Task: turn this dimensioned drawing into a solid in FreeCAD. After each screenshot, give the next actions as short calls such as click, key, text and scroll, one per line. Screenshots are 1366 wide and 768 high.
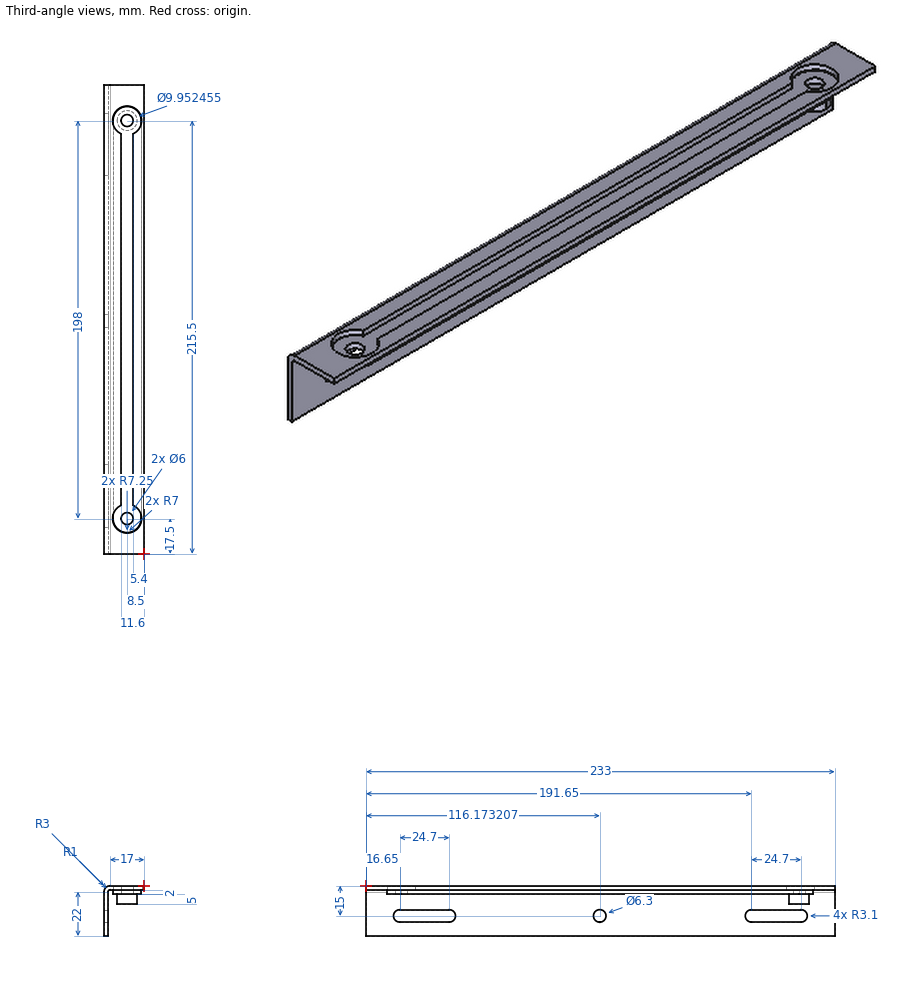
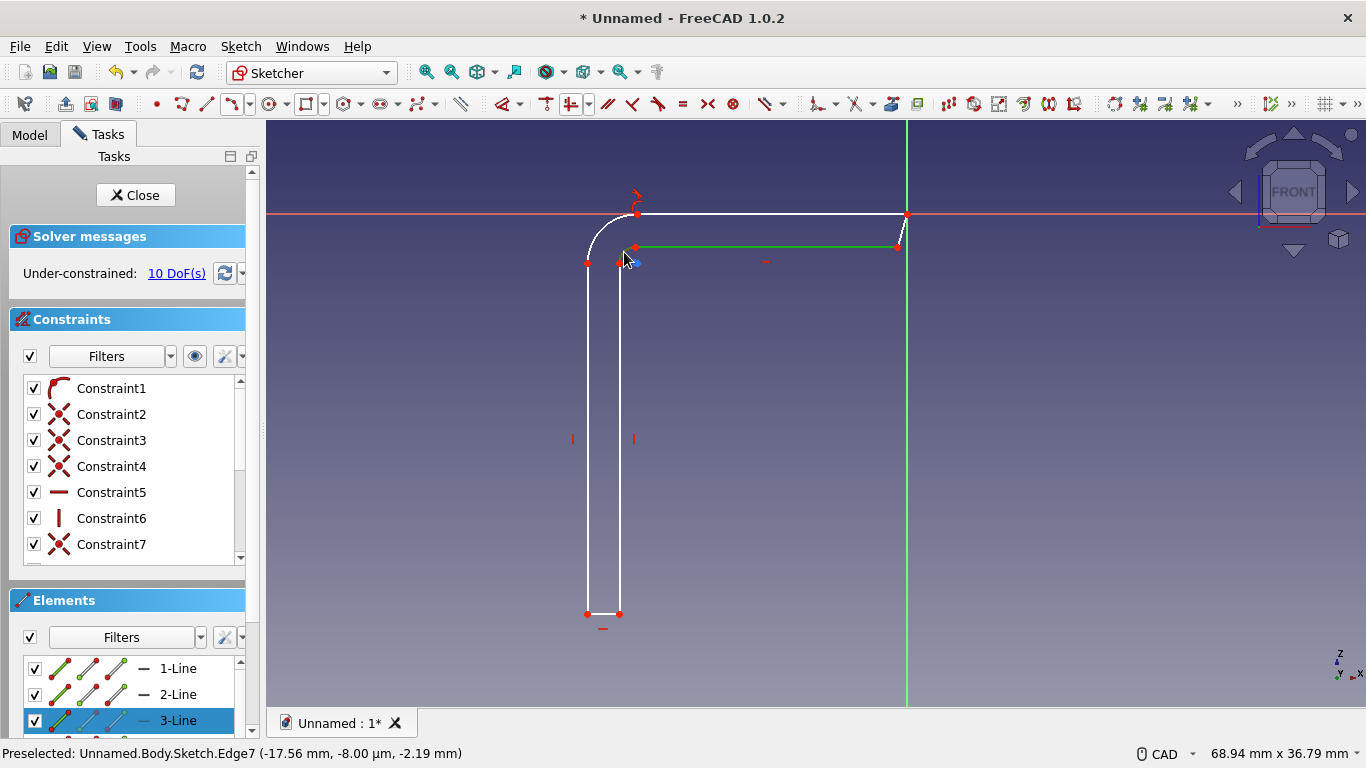
click(658, 104)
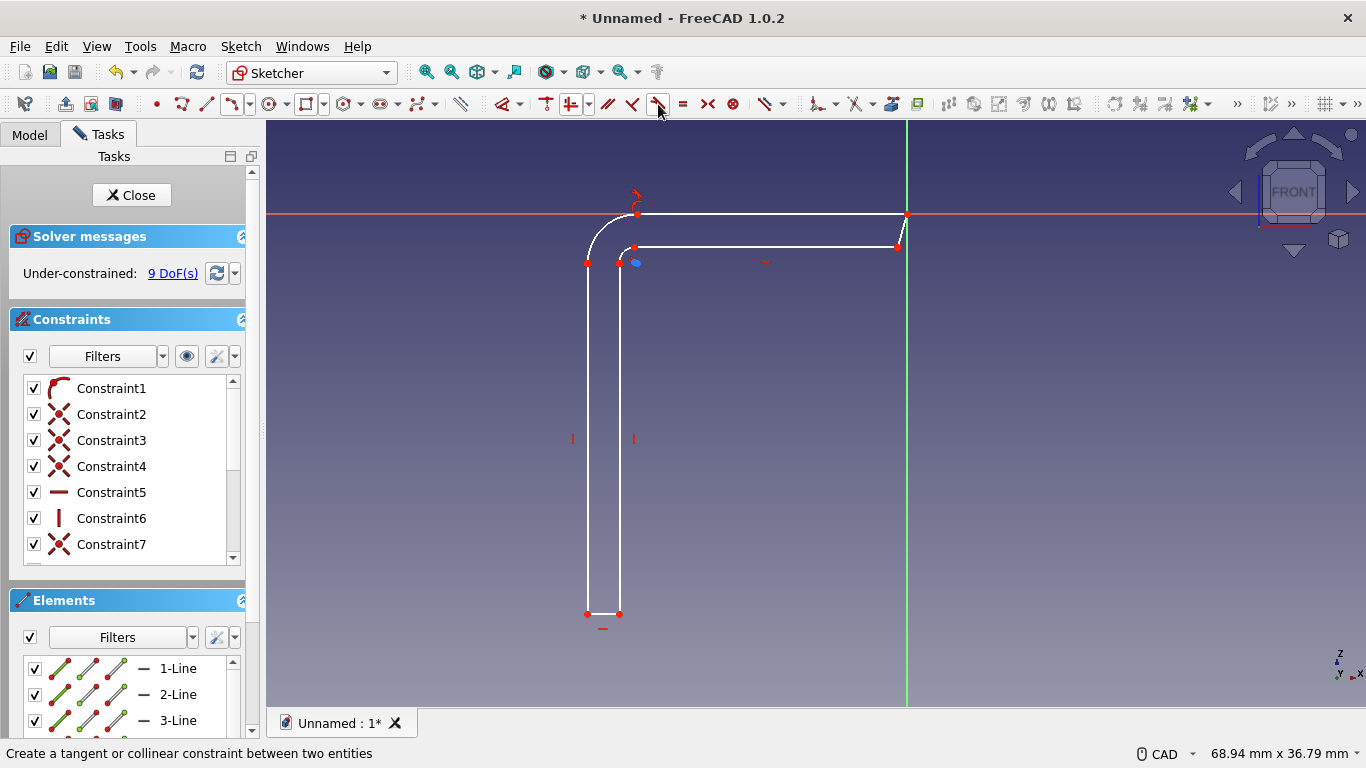
click(620, 369)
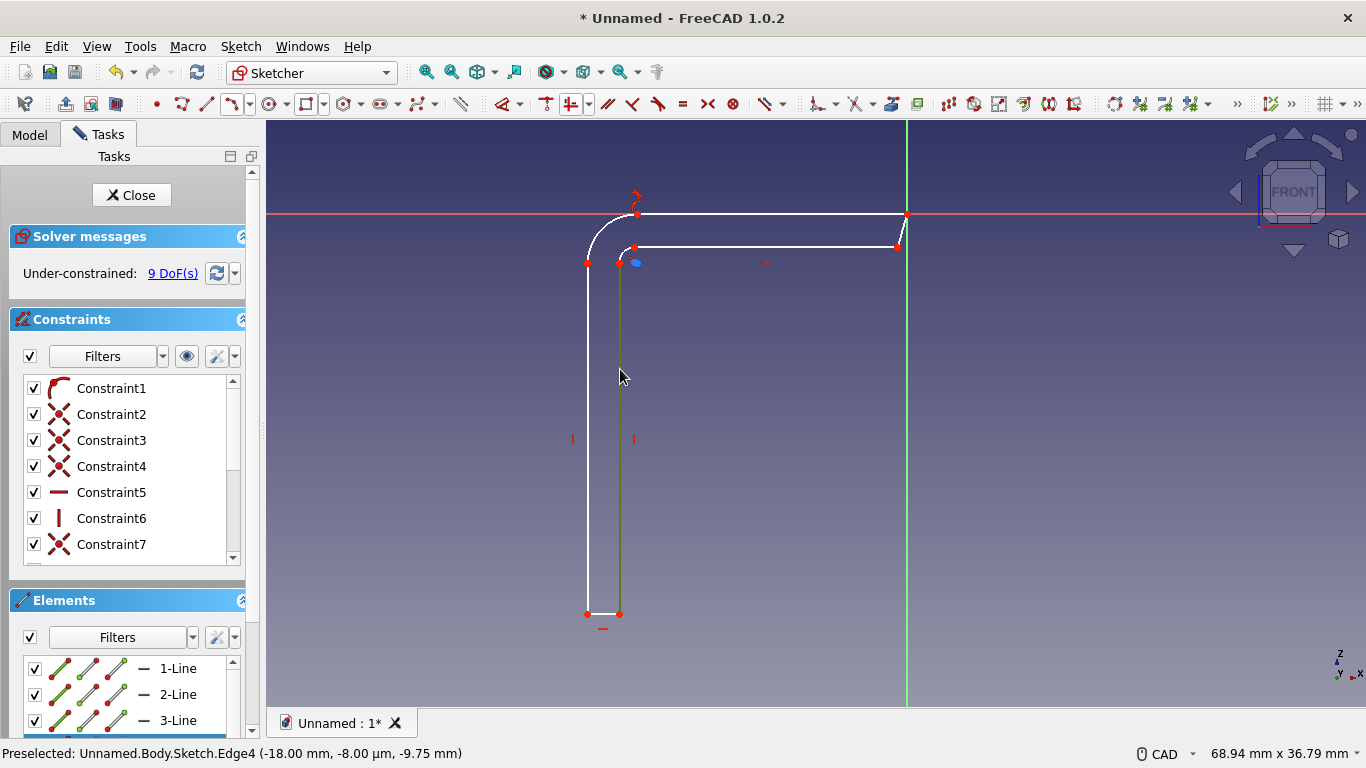
click(624, 252)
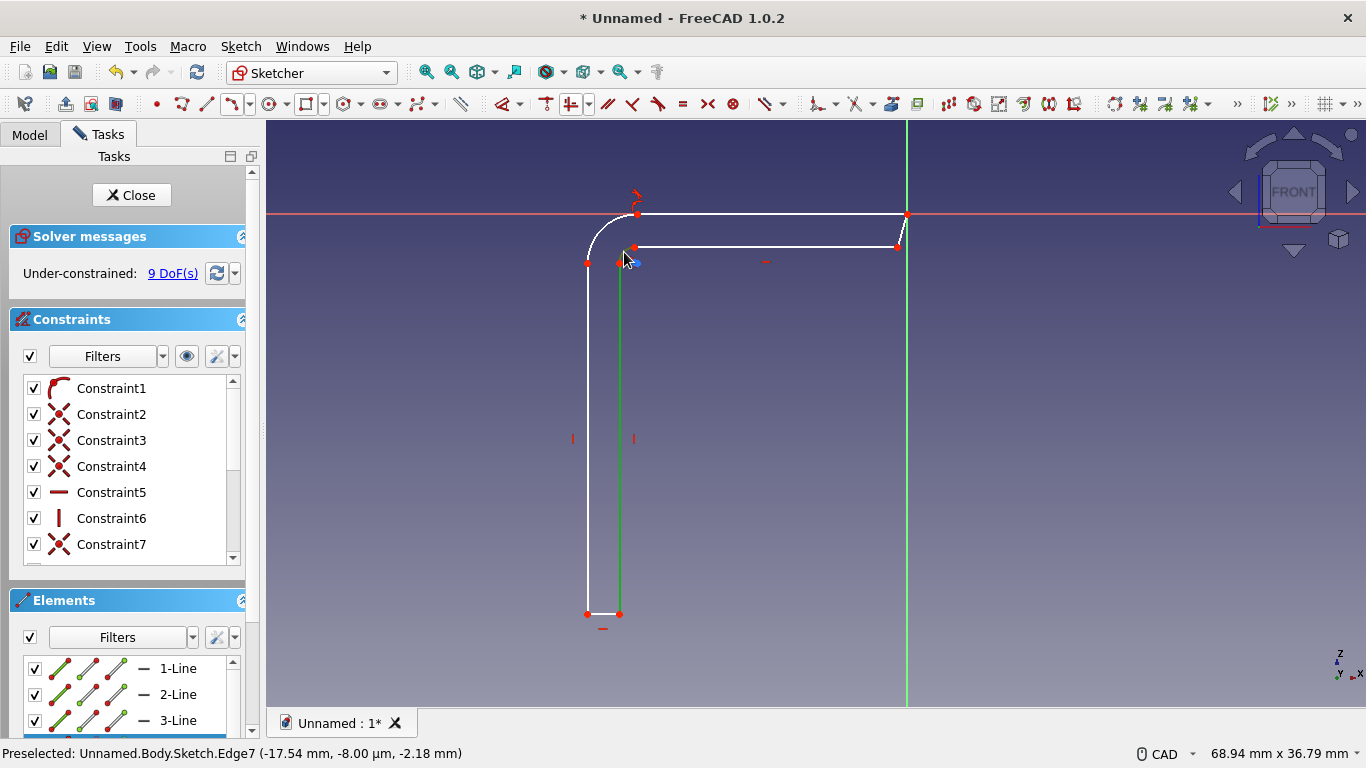
click(658, 104)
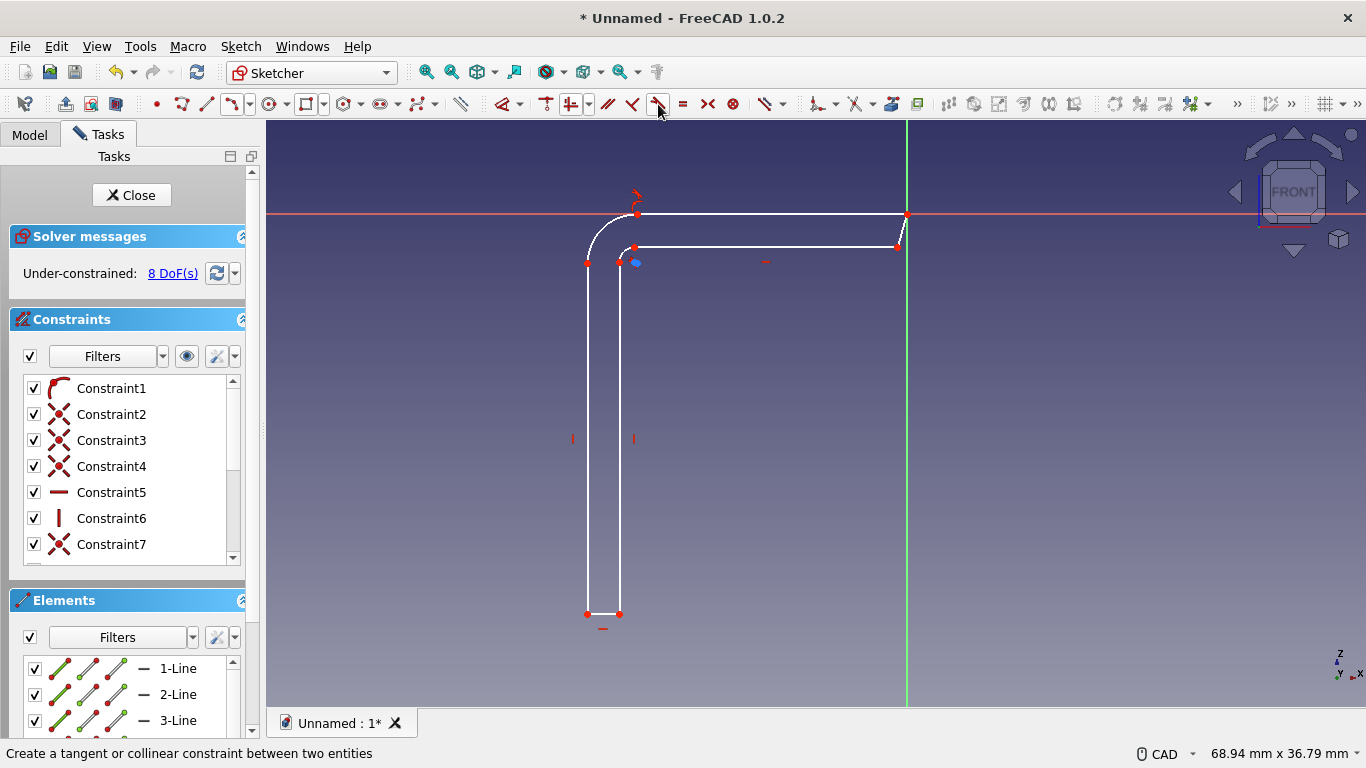
click(588, 509)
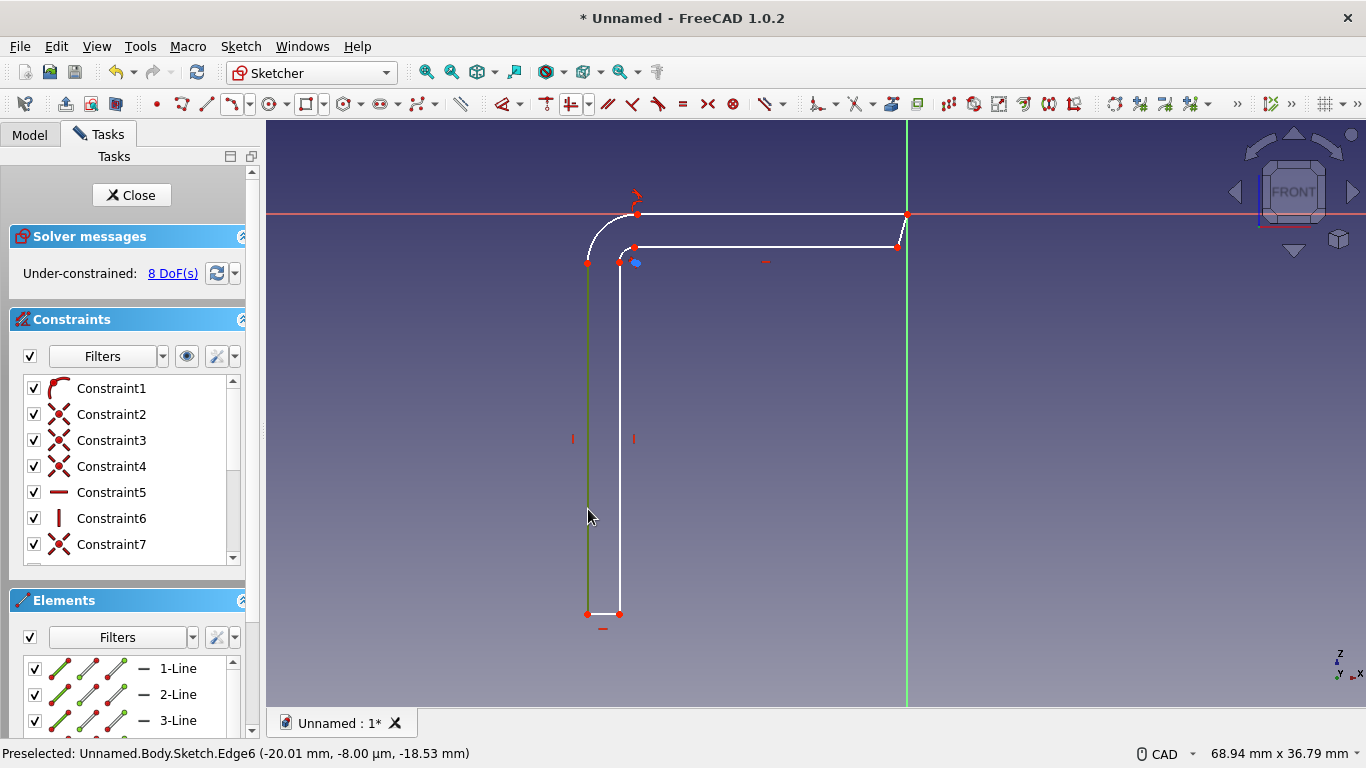
click(593, 241)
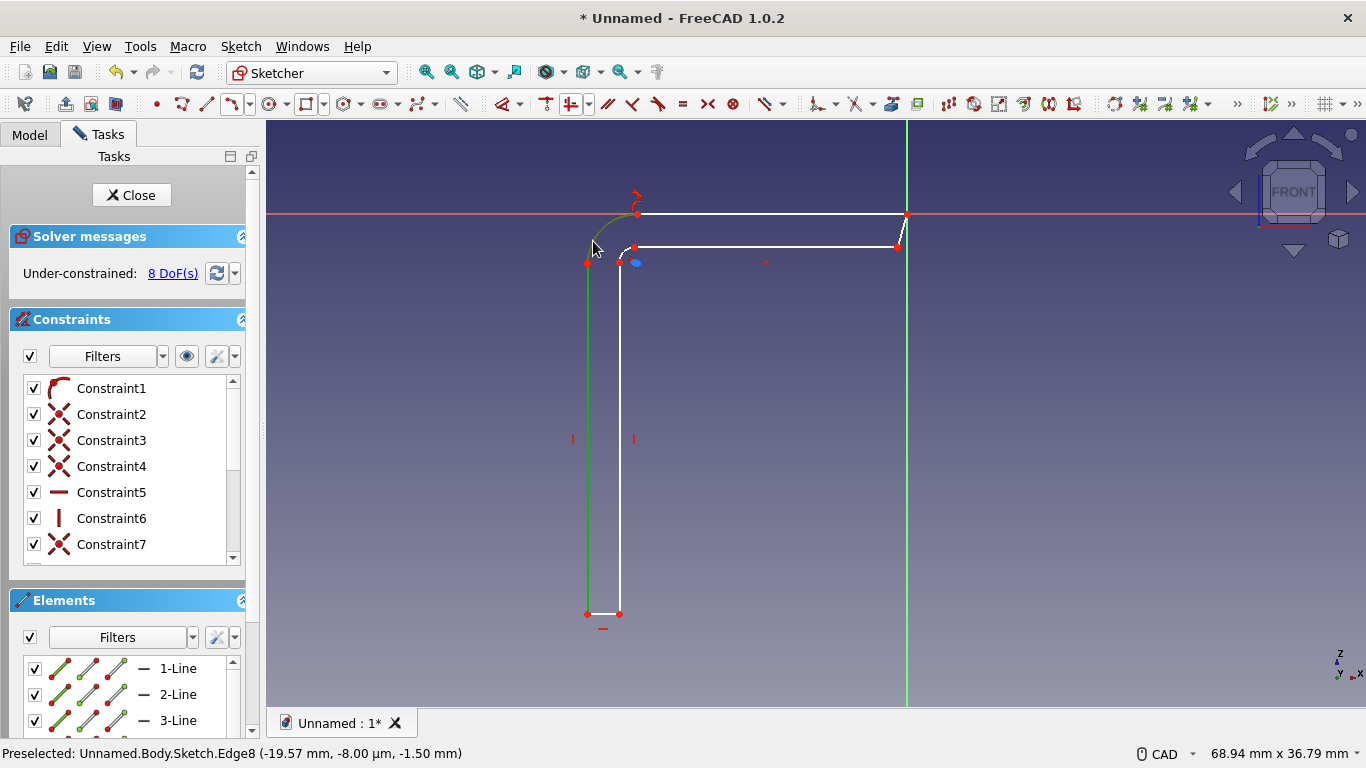
click(658, 104)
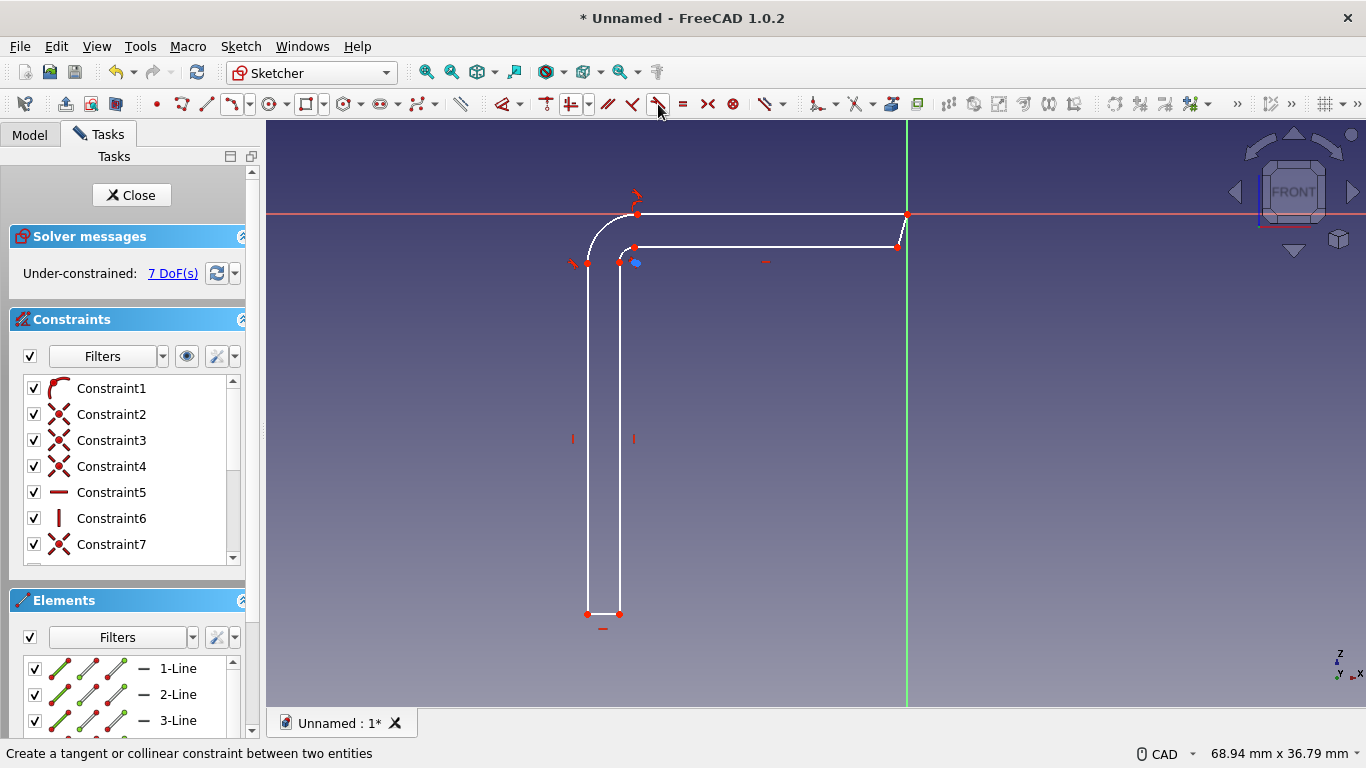
scroll(904, 224, up, 2)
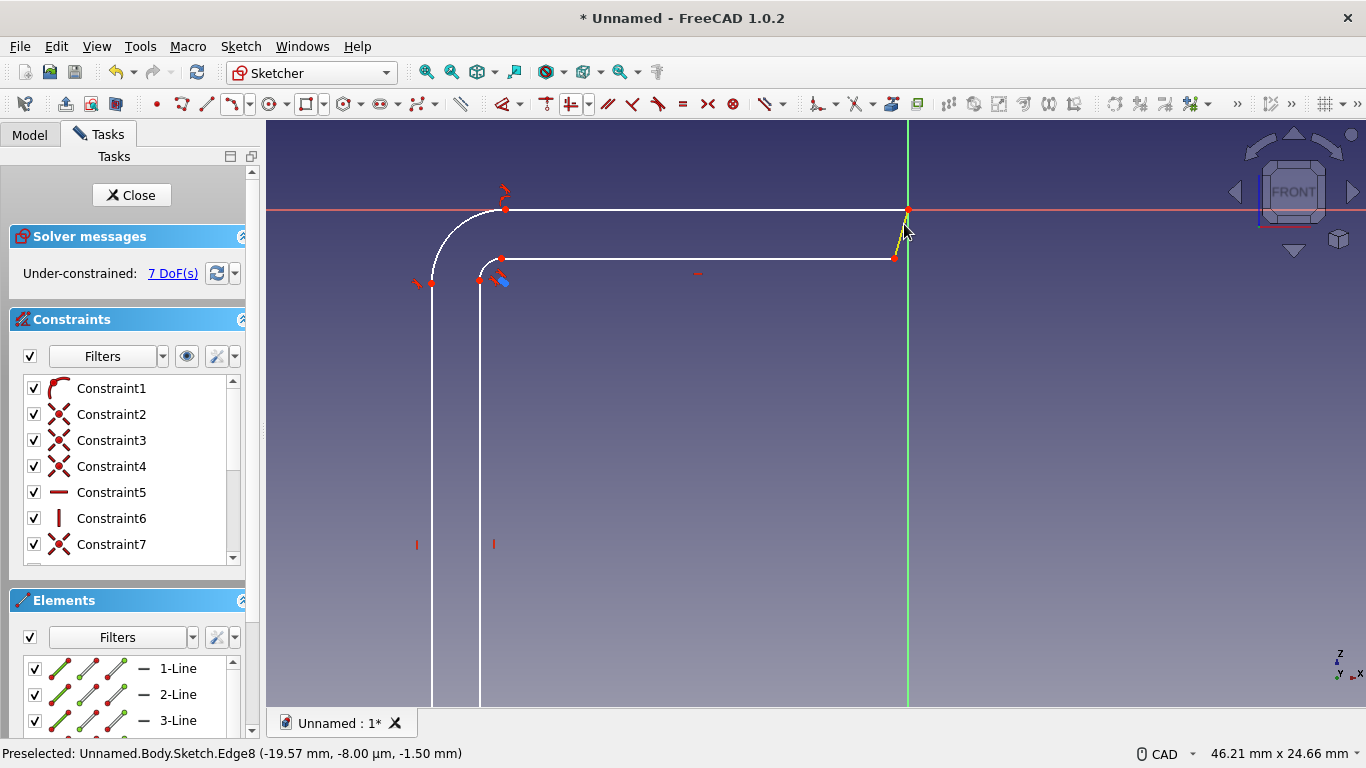
click(904, 224)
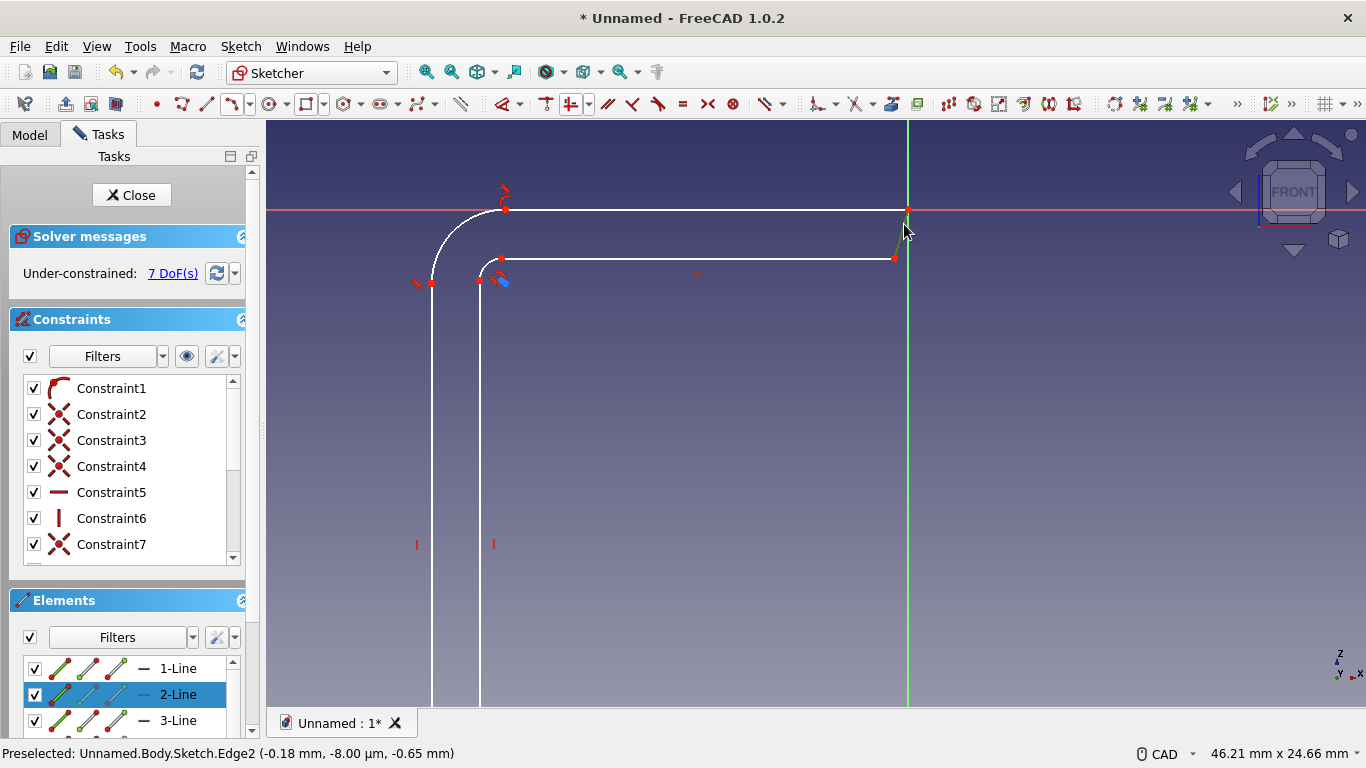
click(588, 104)